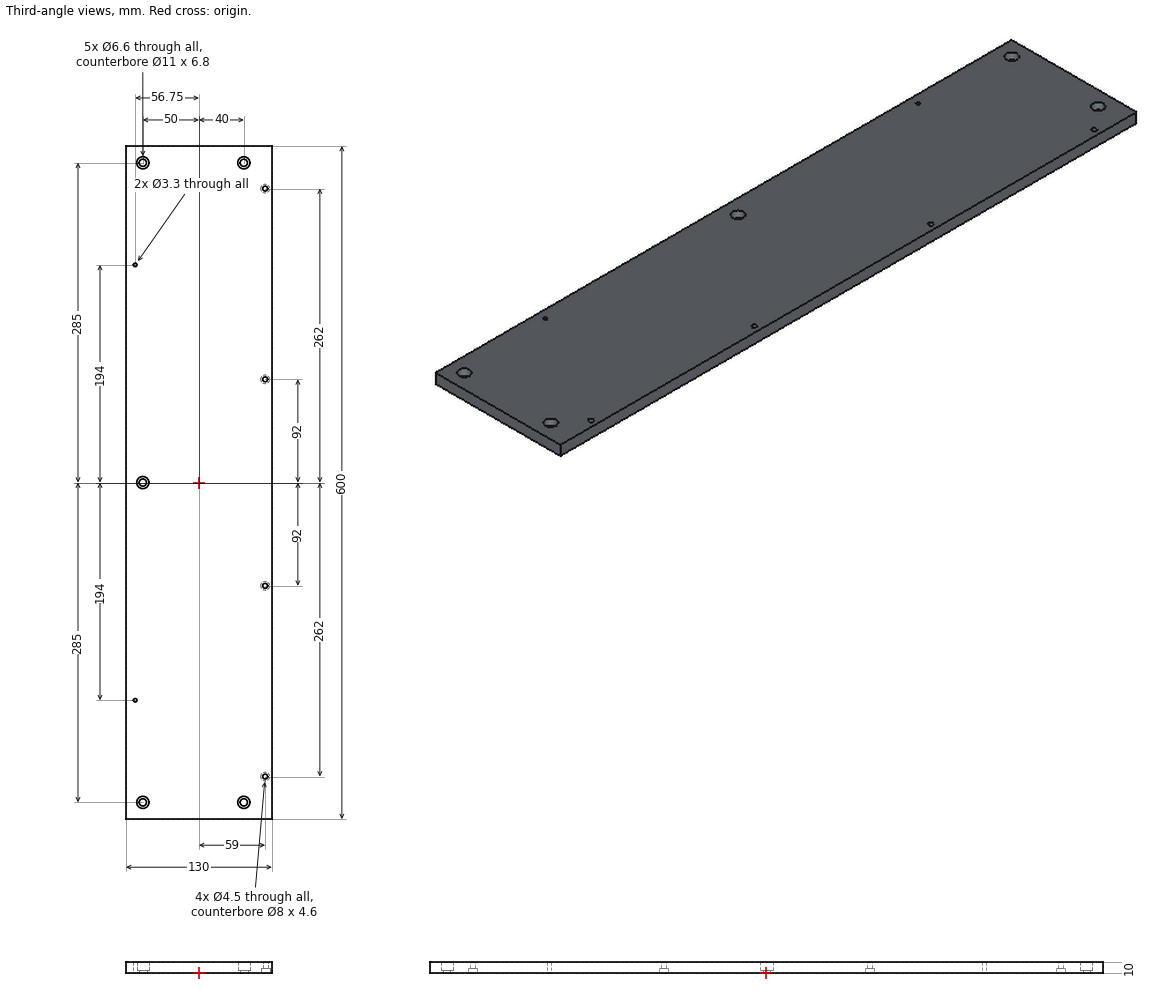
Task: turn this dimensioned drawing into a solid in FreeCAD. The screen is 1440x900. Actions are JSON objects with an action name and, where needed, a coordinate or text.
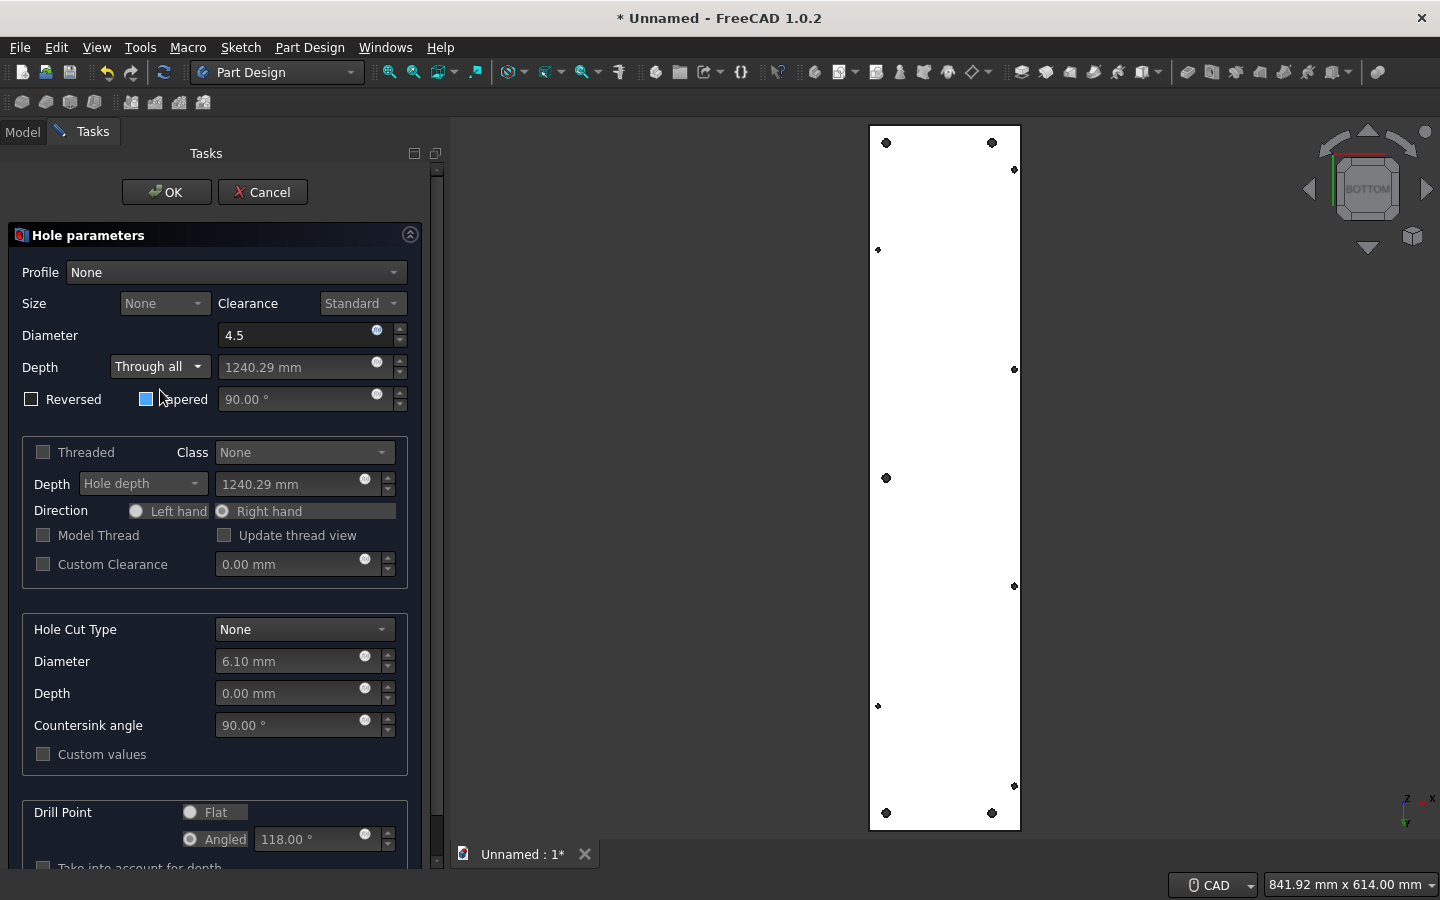
{"action": "left_click", "coordinate": [306, 630]}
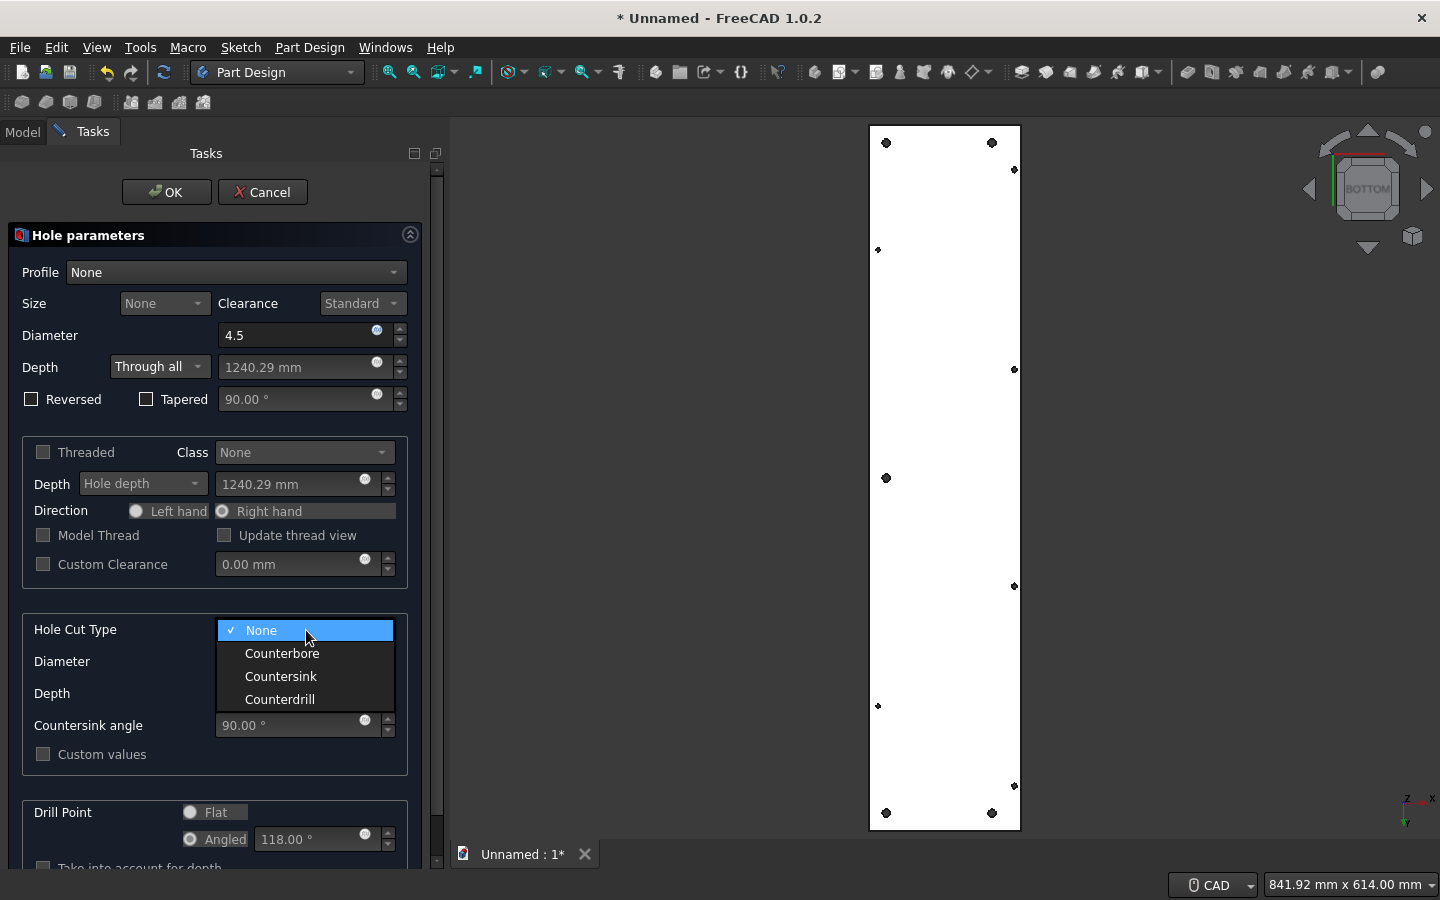
{"action": "left_click", "coordinate": [304, 654]}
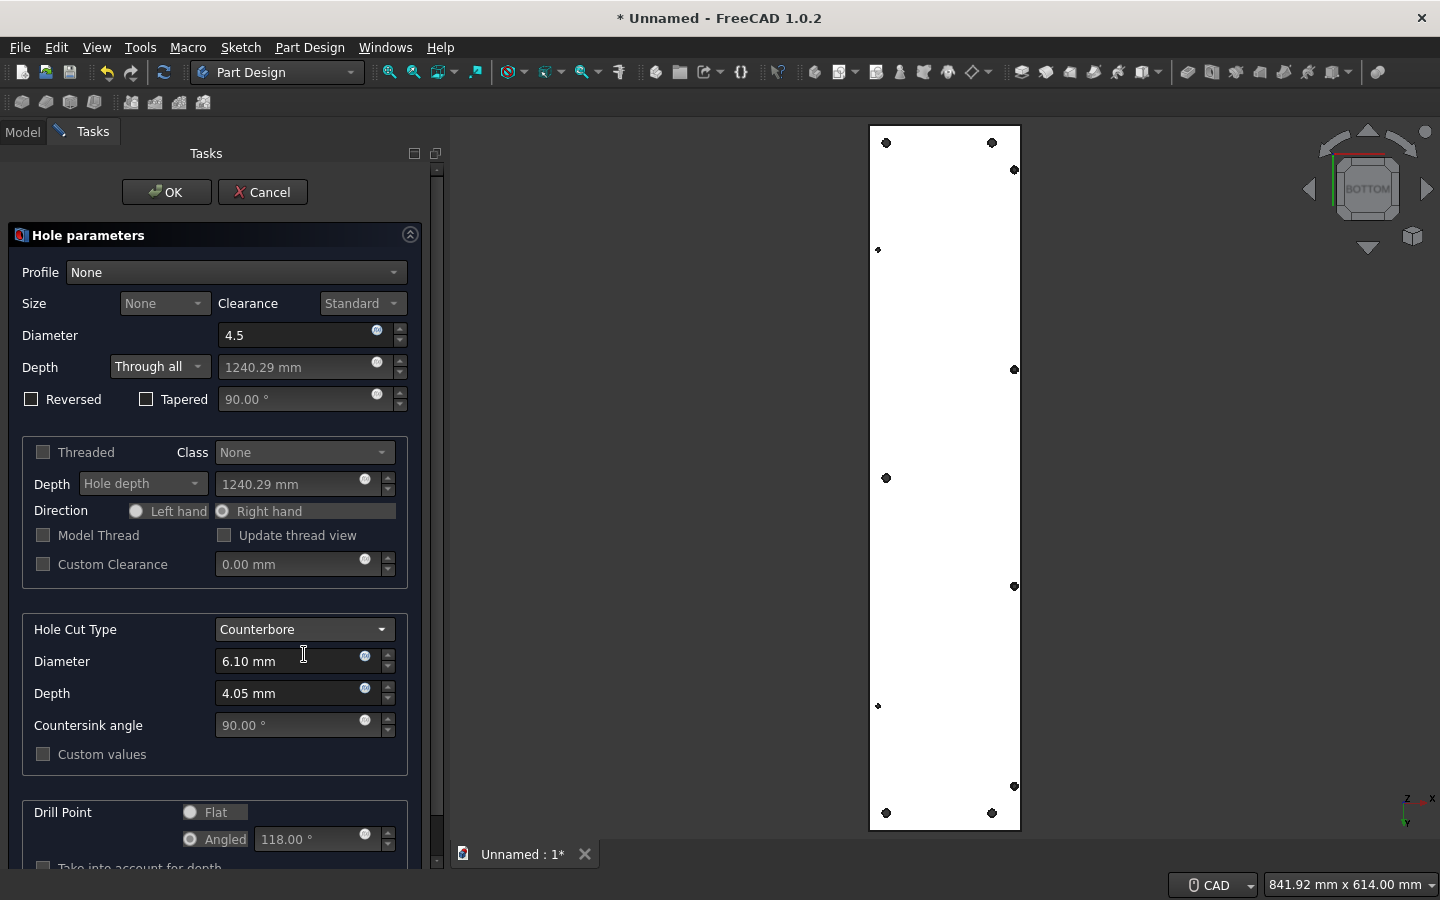
{"action": "triple_click", "coordinate": [298, 661]}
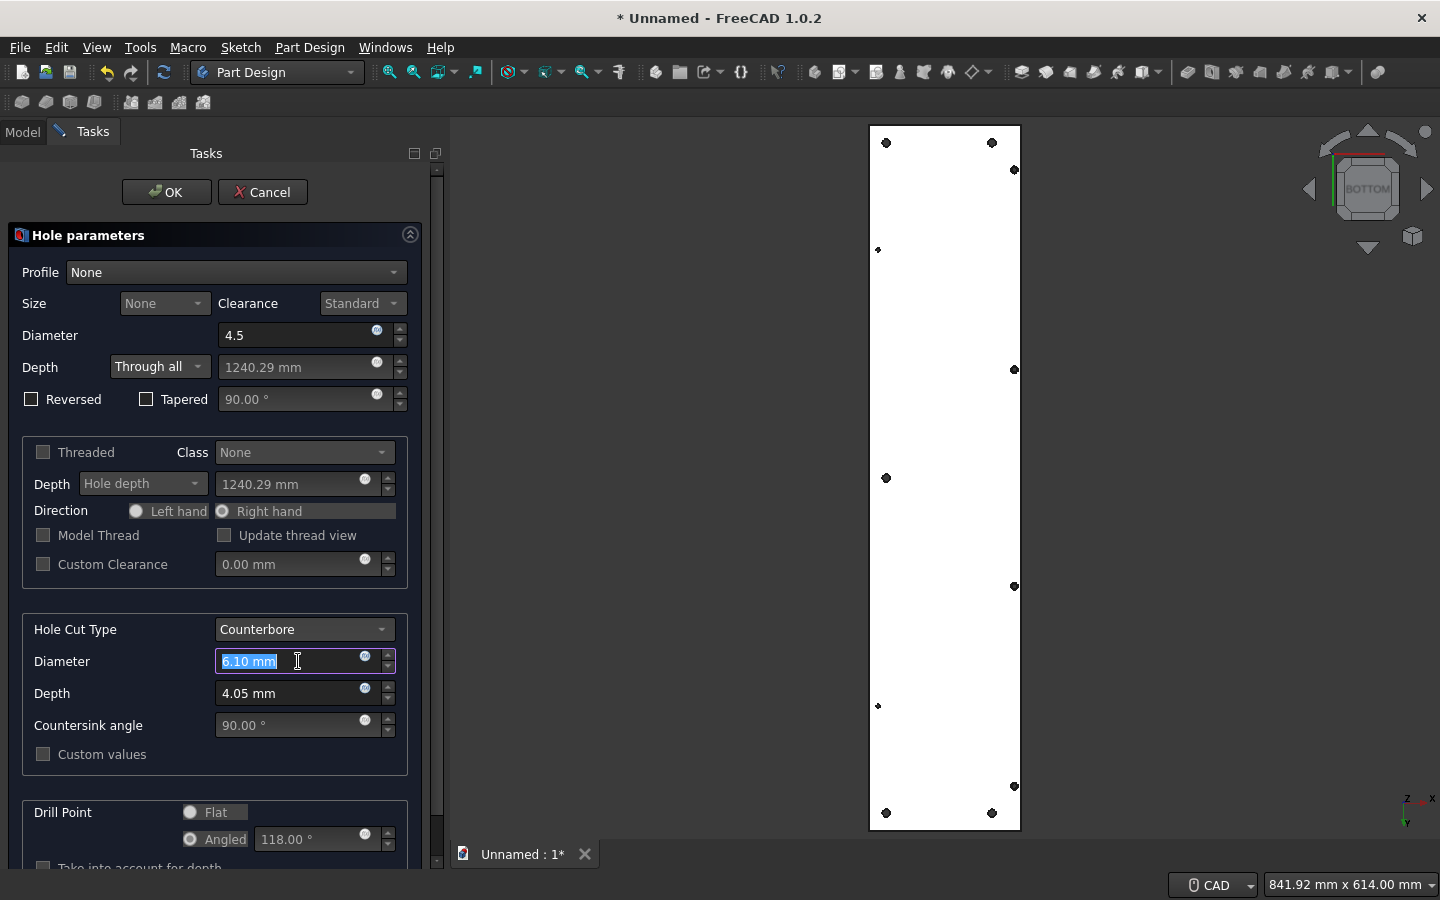
{"action": "type", "text": "8"}
{"action": "key", "text": "Tab"}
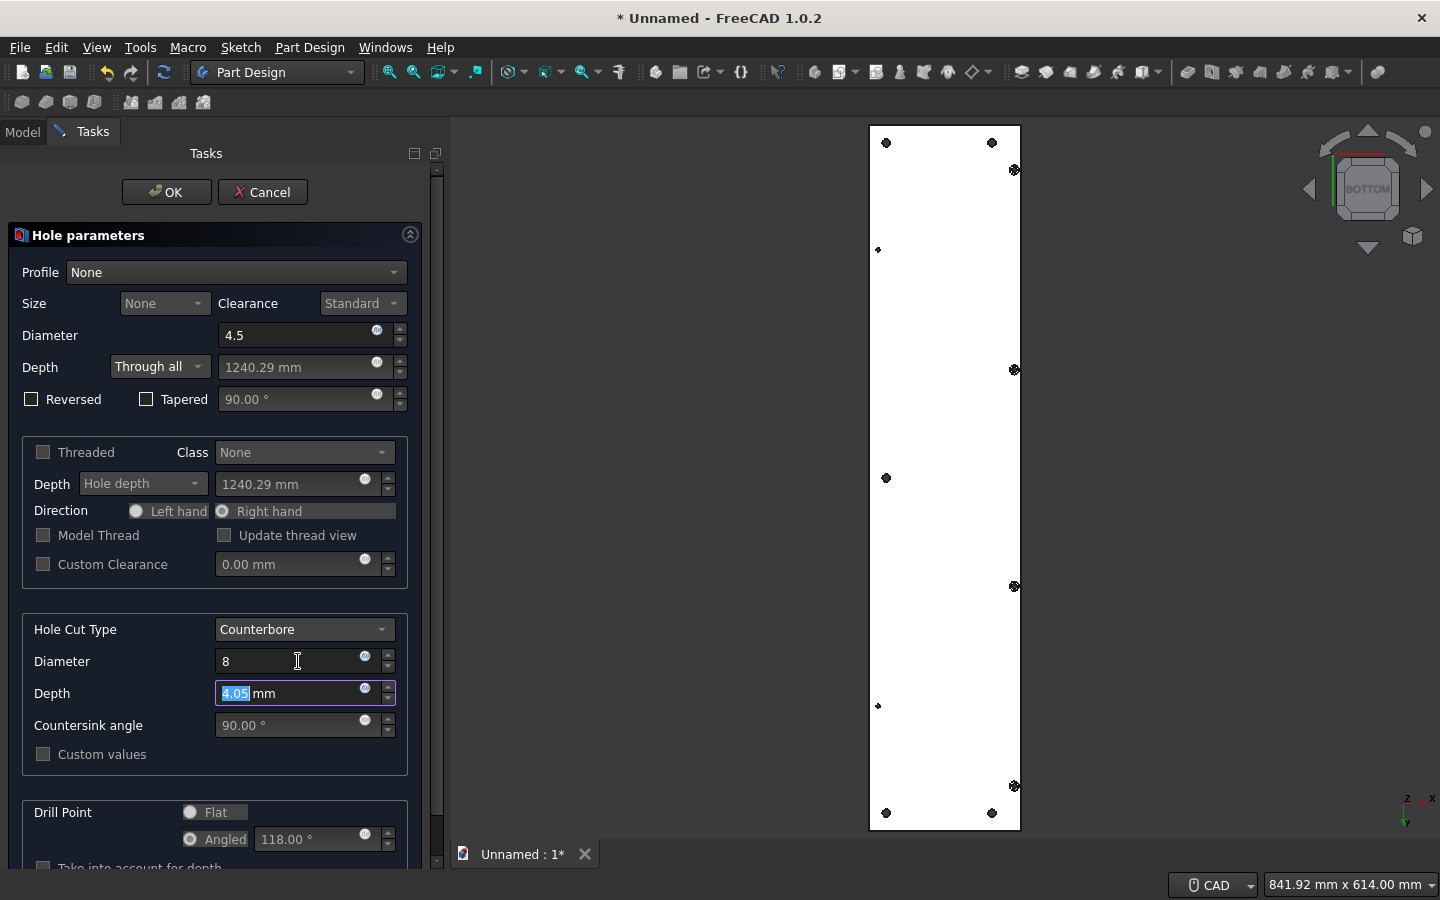
{"action": "type", "text": "4.6"}
{"action": "key", "text": "Tab"}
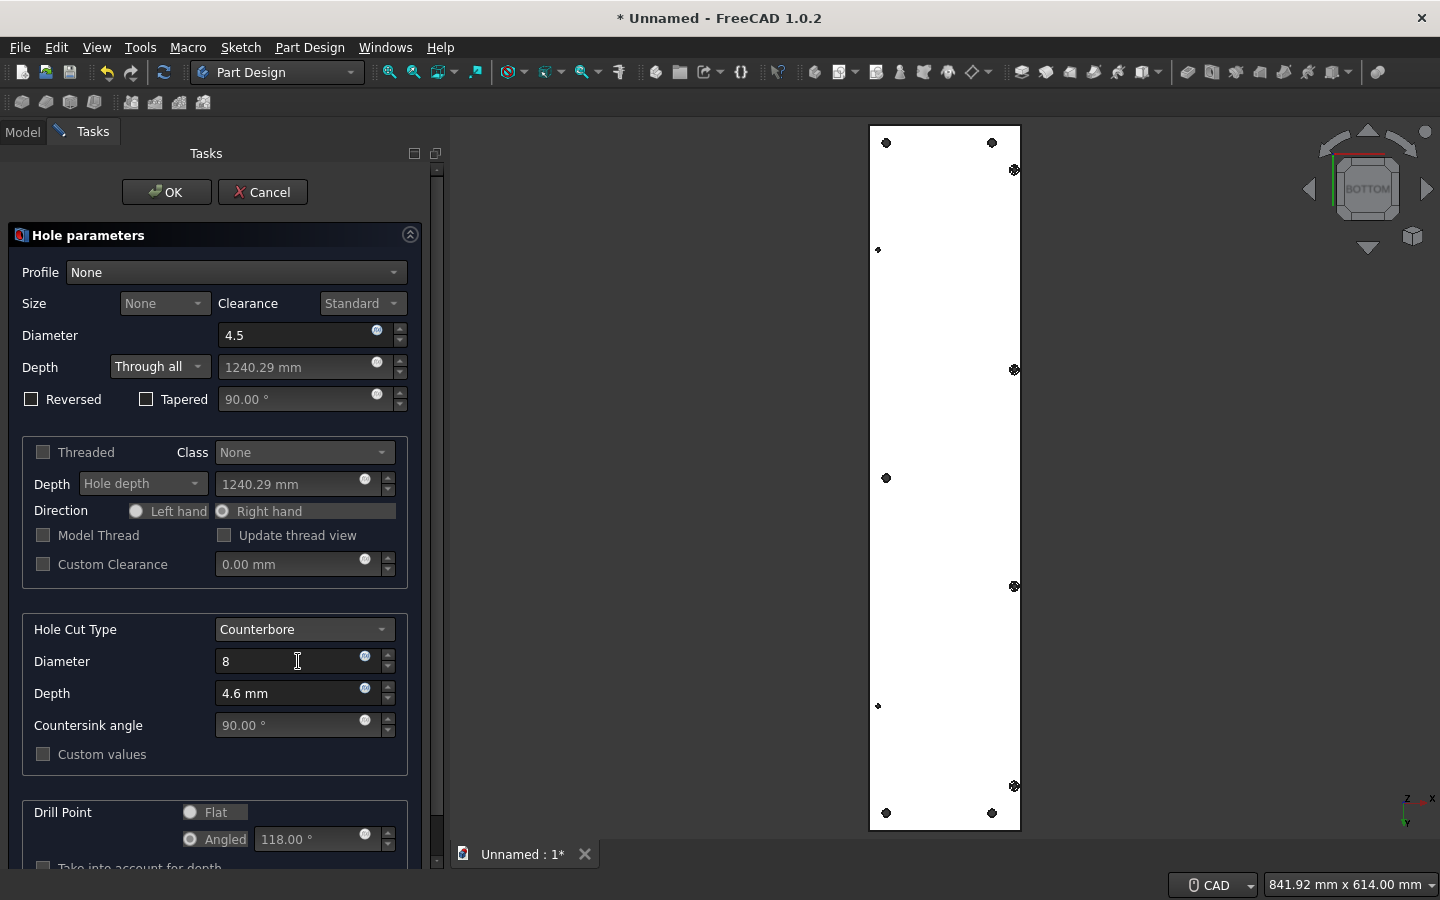
{"action": "left_click", "coordinate": [167, 192]}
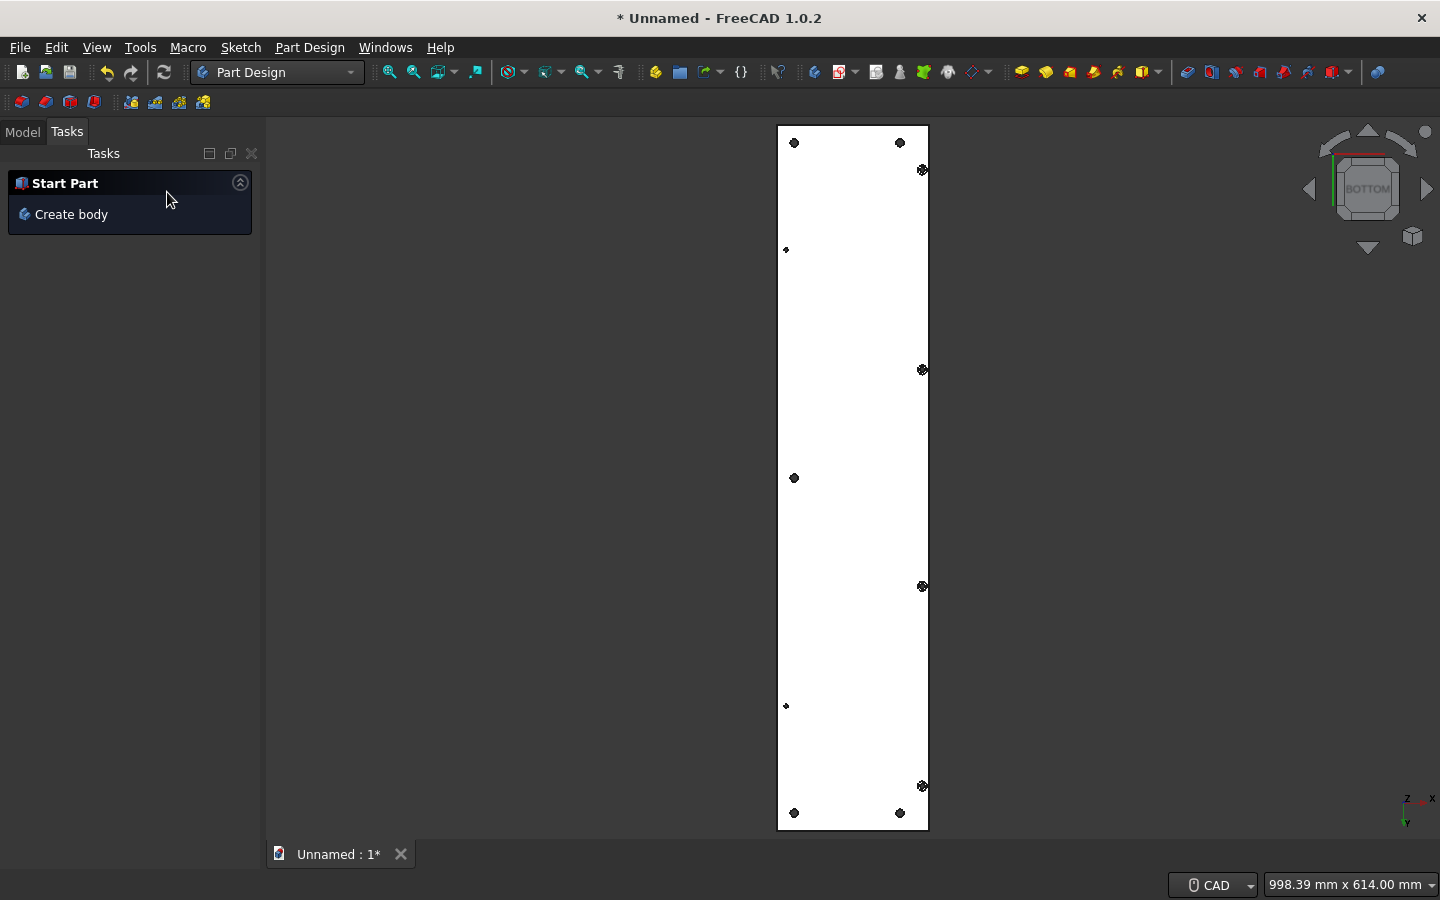
{"action": "key", "text": "0"}